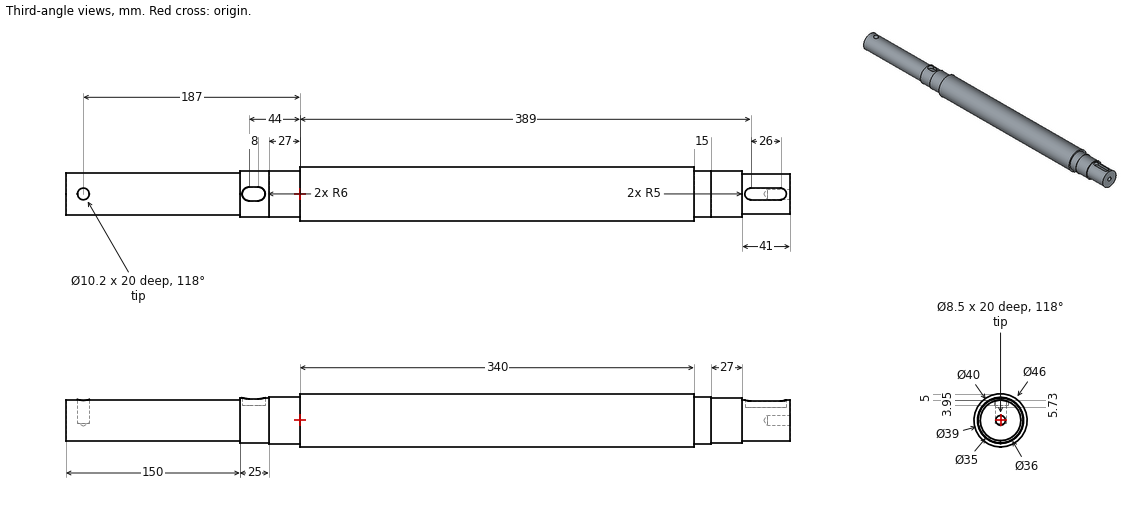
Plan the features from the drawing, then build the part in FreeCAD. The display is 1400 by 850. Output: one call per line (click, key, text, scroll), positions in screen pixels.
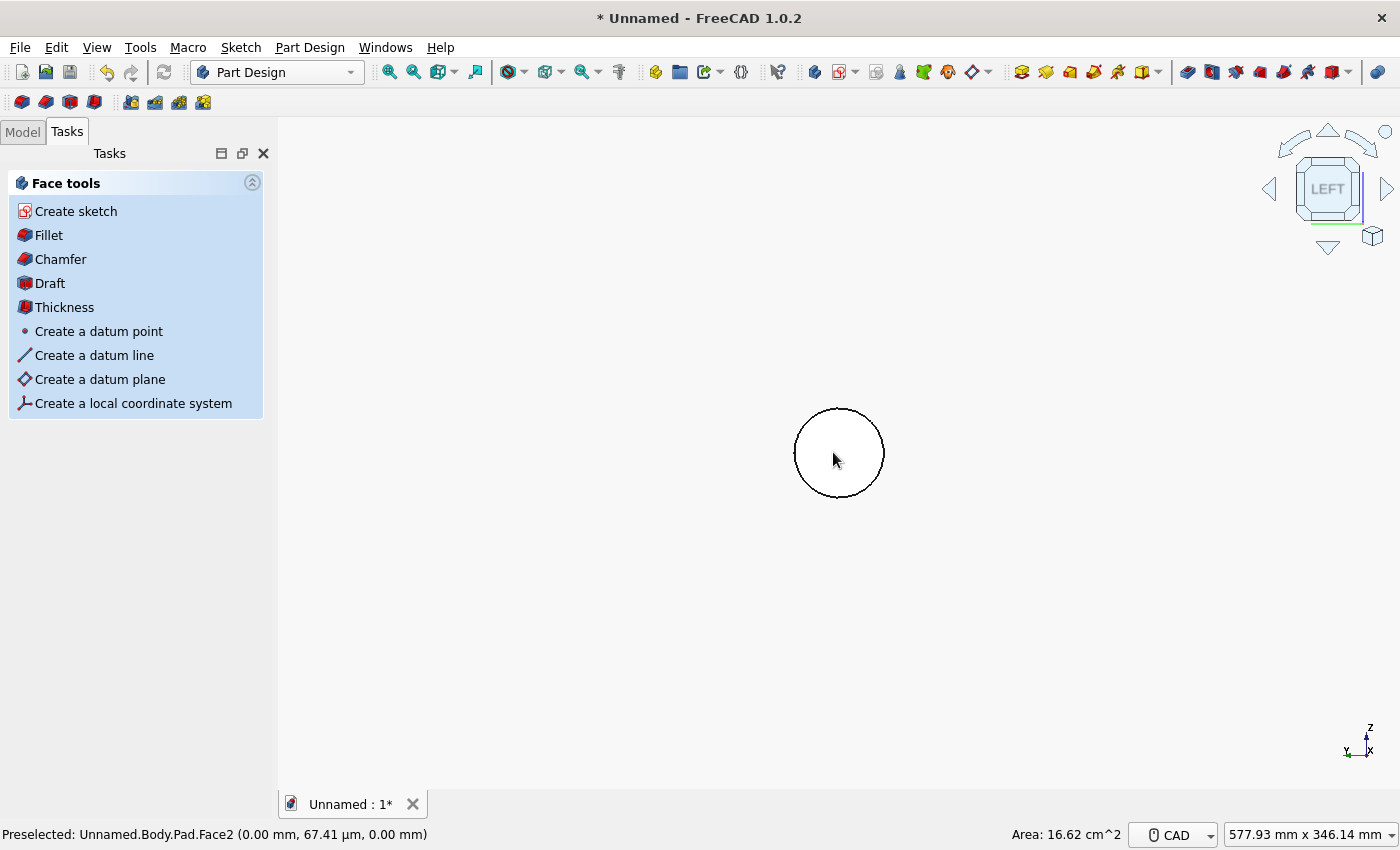
click(840, 72)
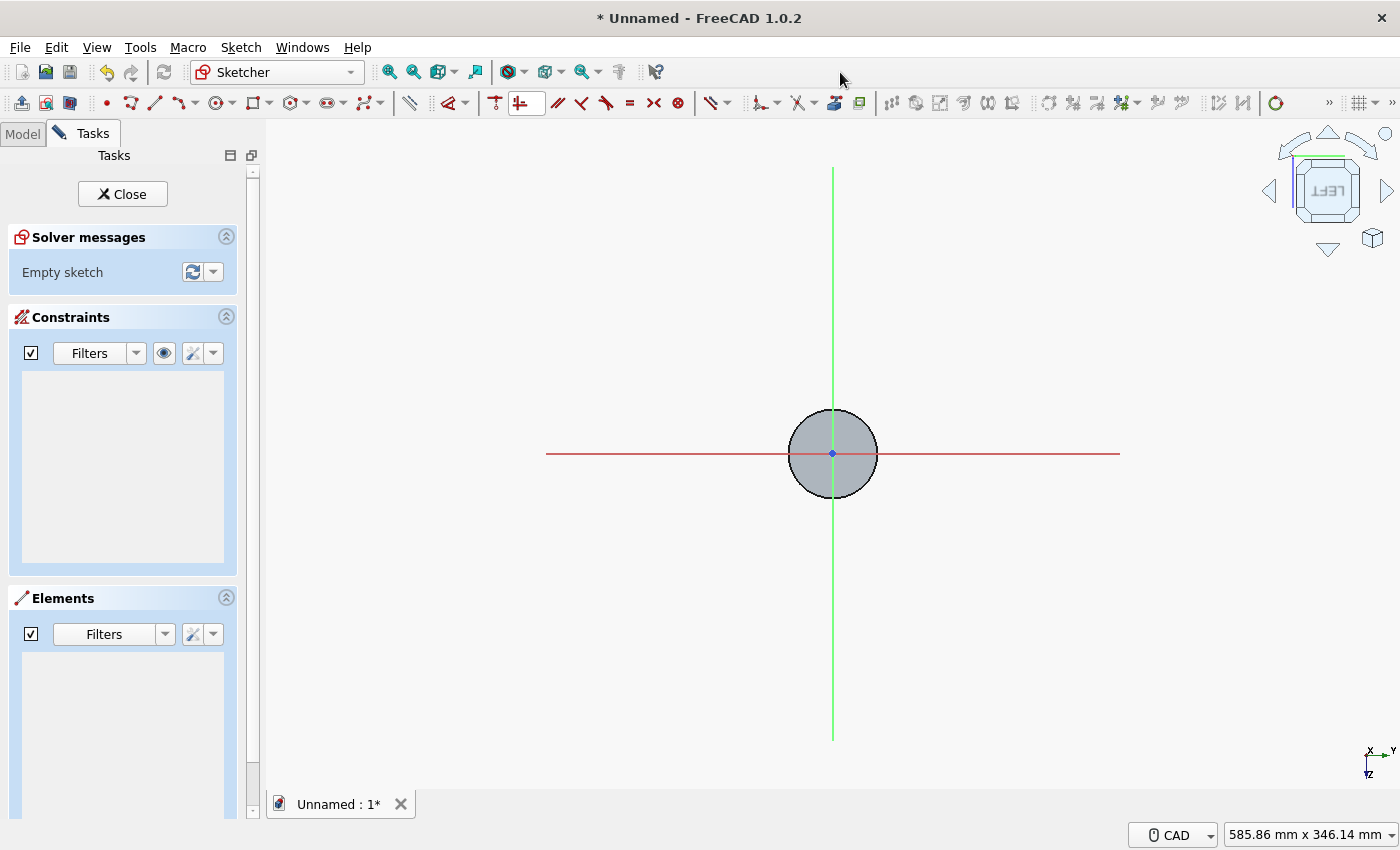
scroll(846, 454, up, 9)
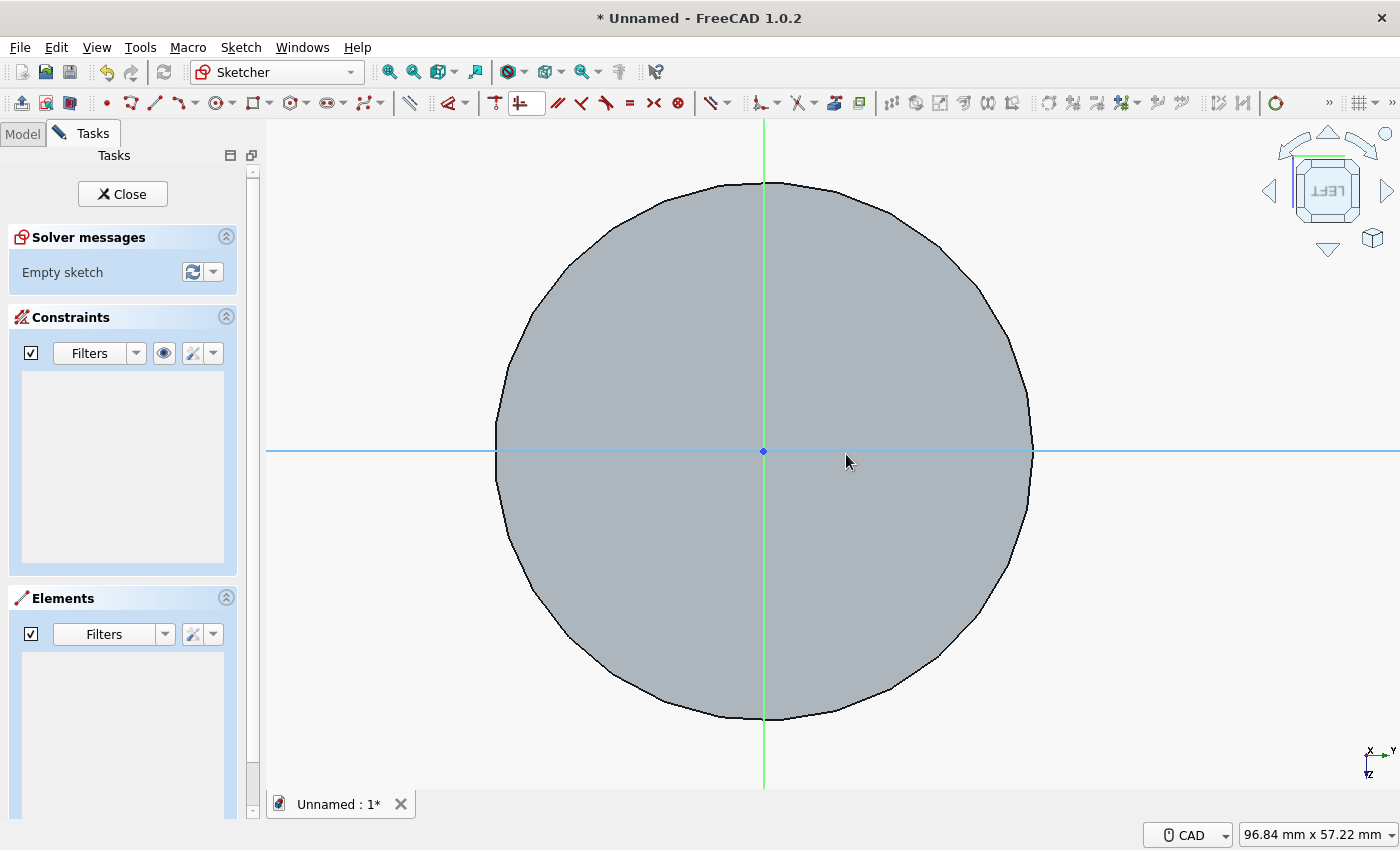
click(216, 104)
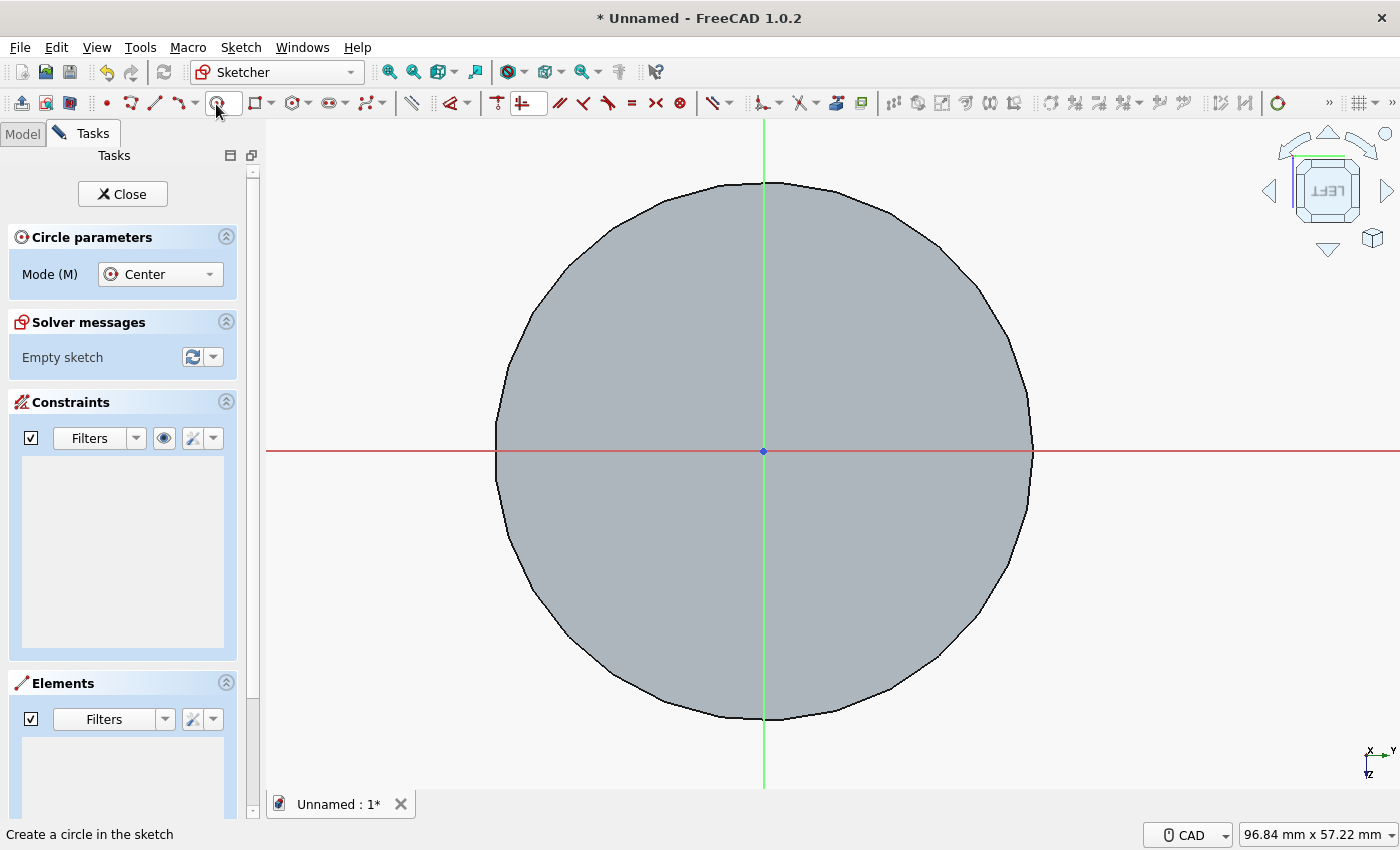
click(764, 451)
click(930, 286)
key(Escape)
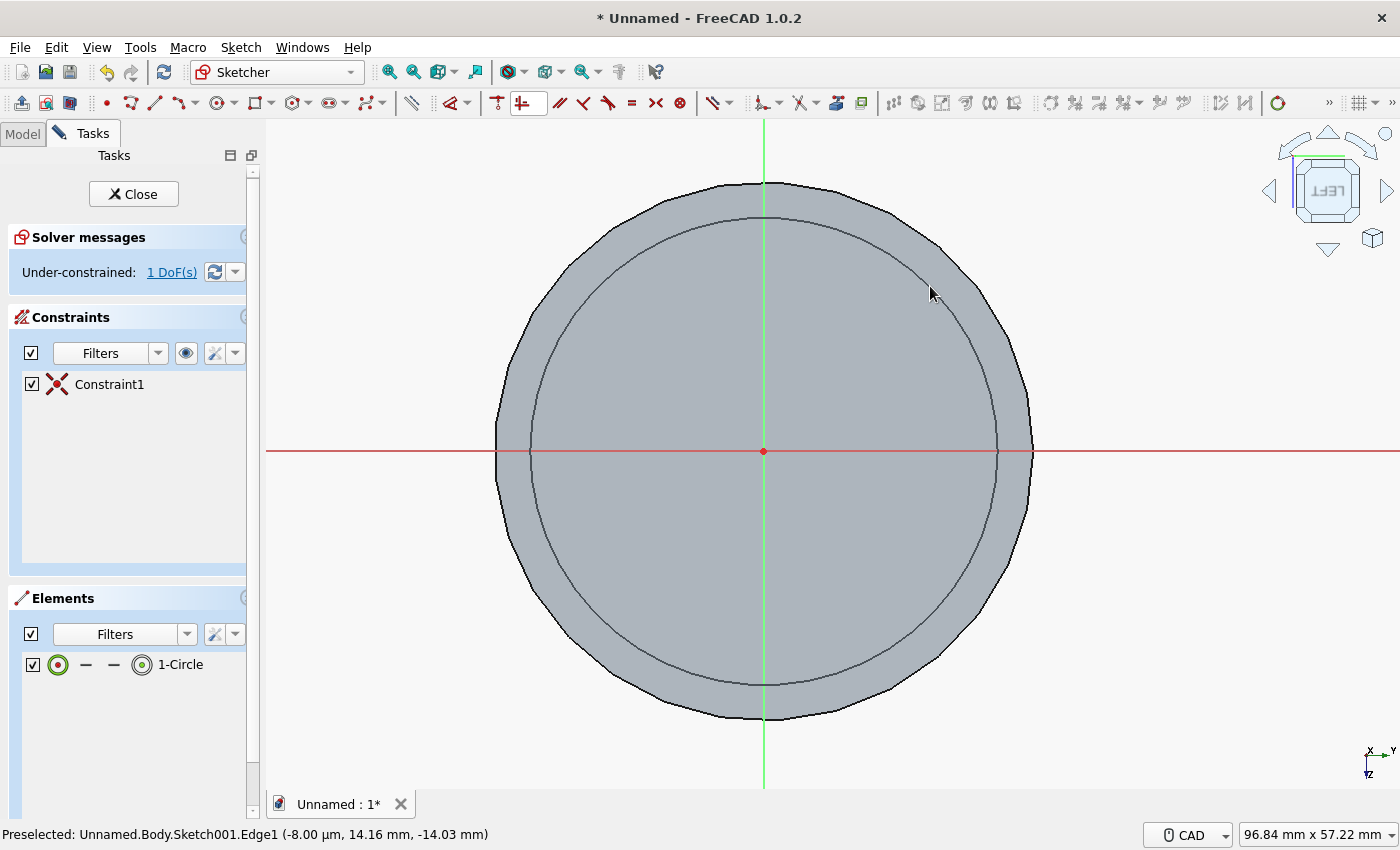
click(450, 104)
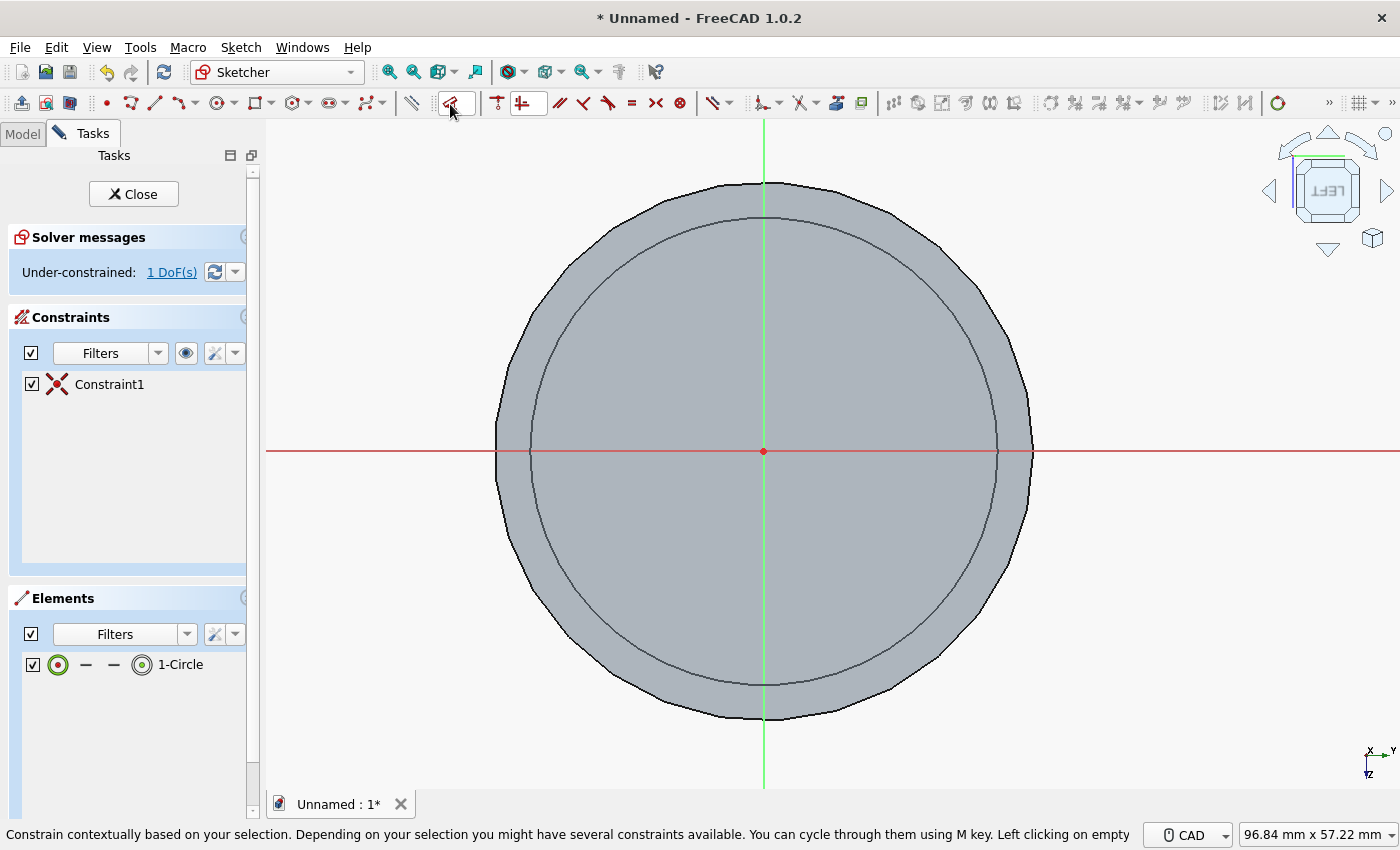
click(929, 286)
click(952, 263)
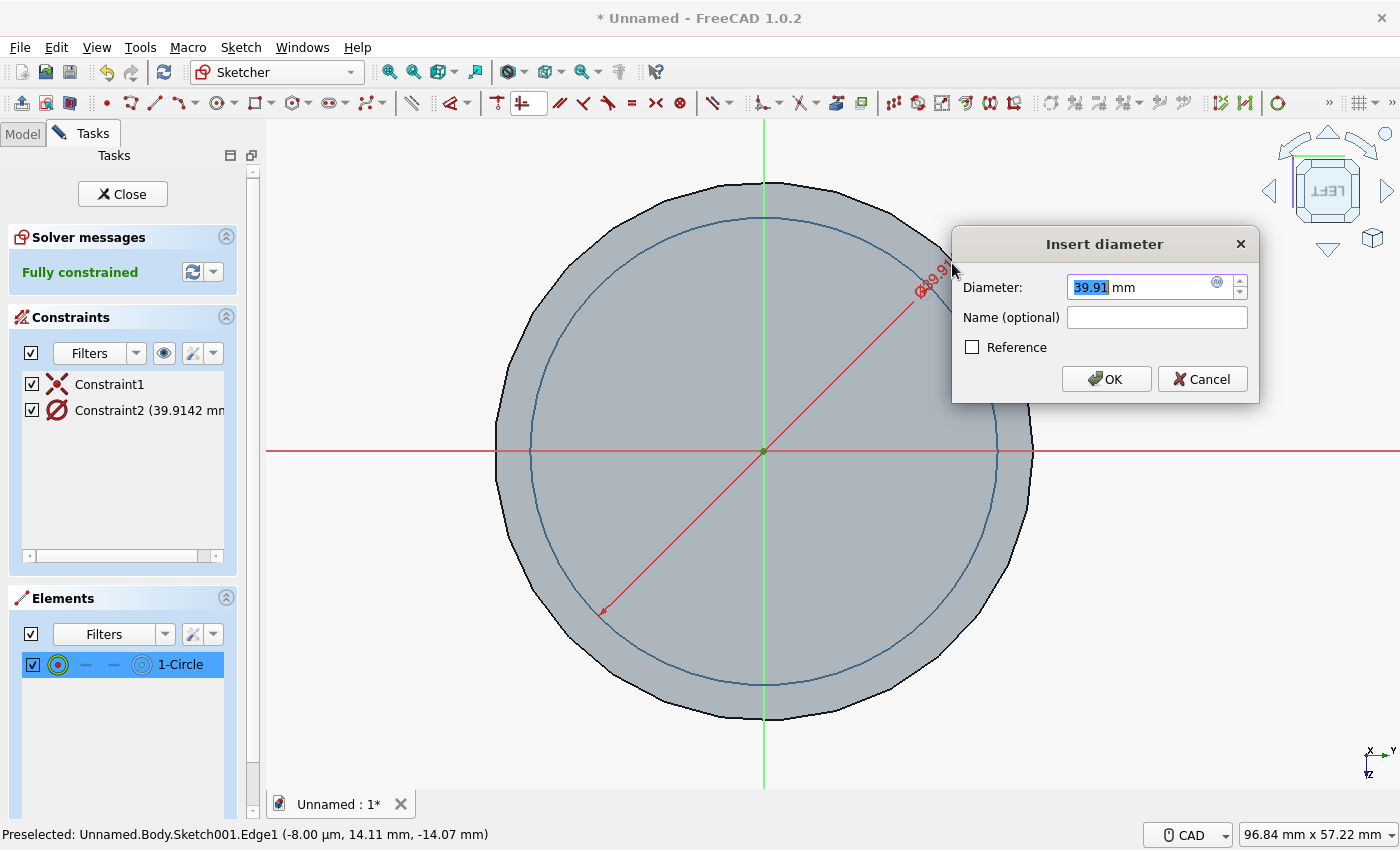
text(40)
key(Return)
key(Escape)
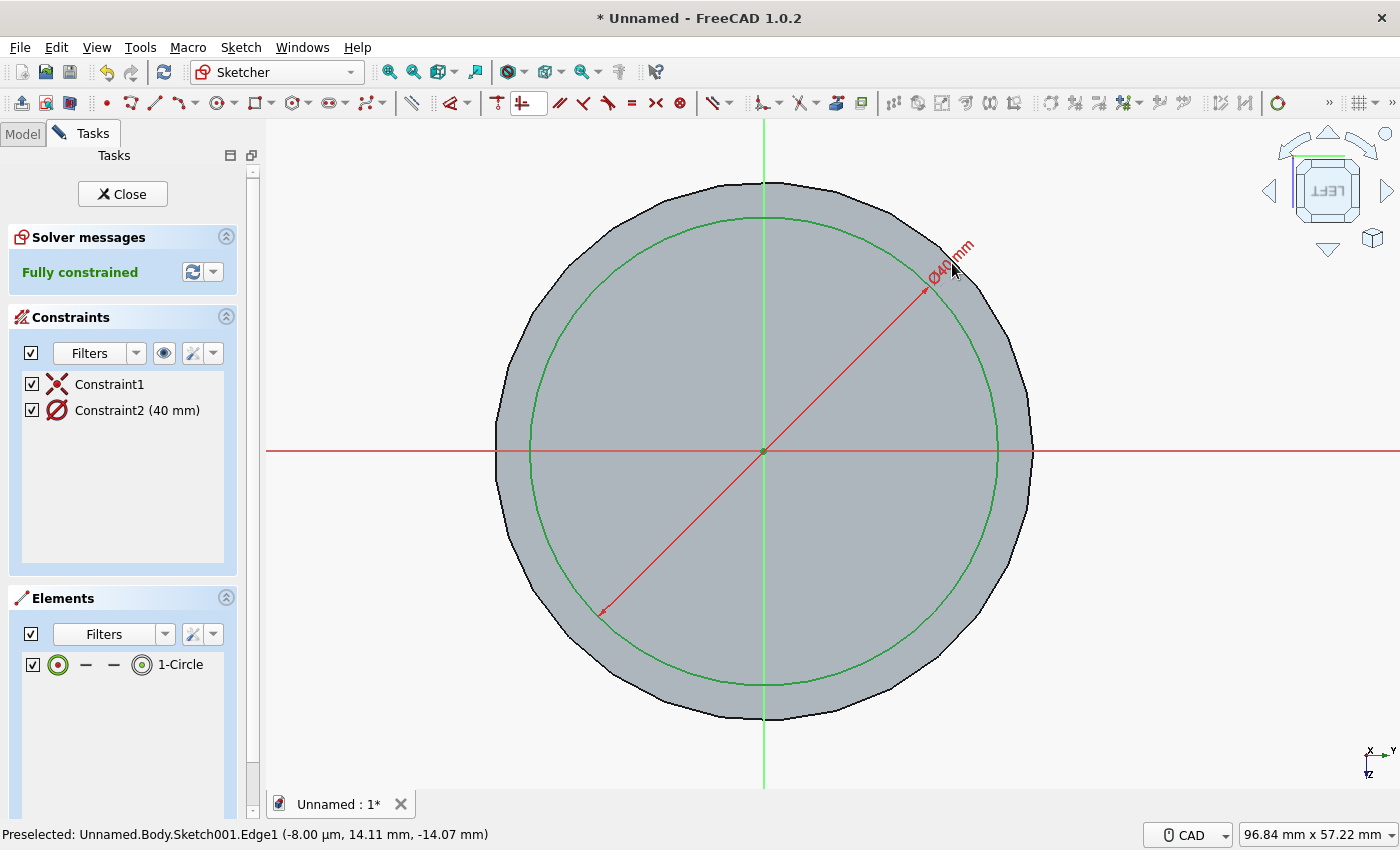
click(123, 194)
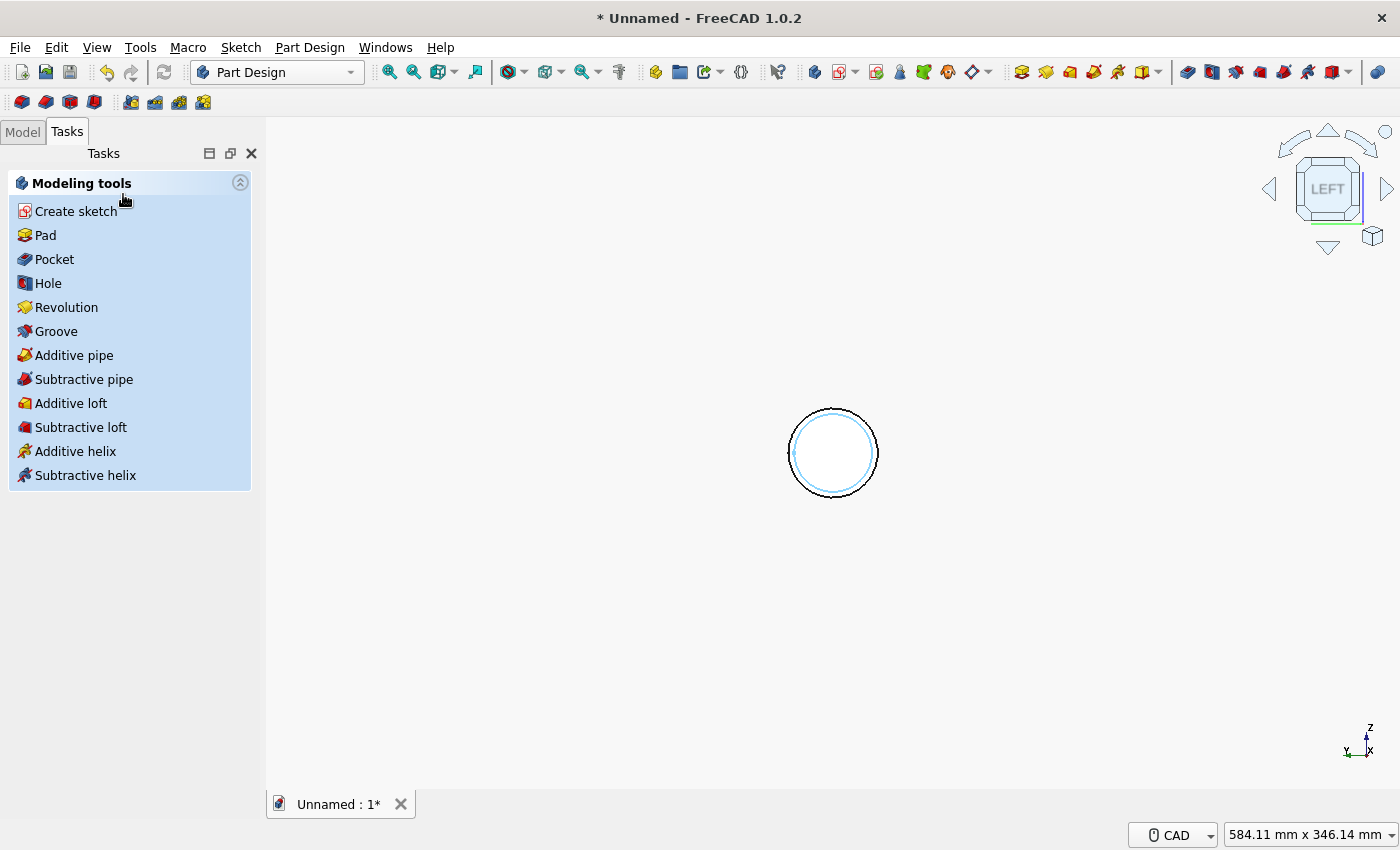
click(1022, 72)